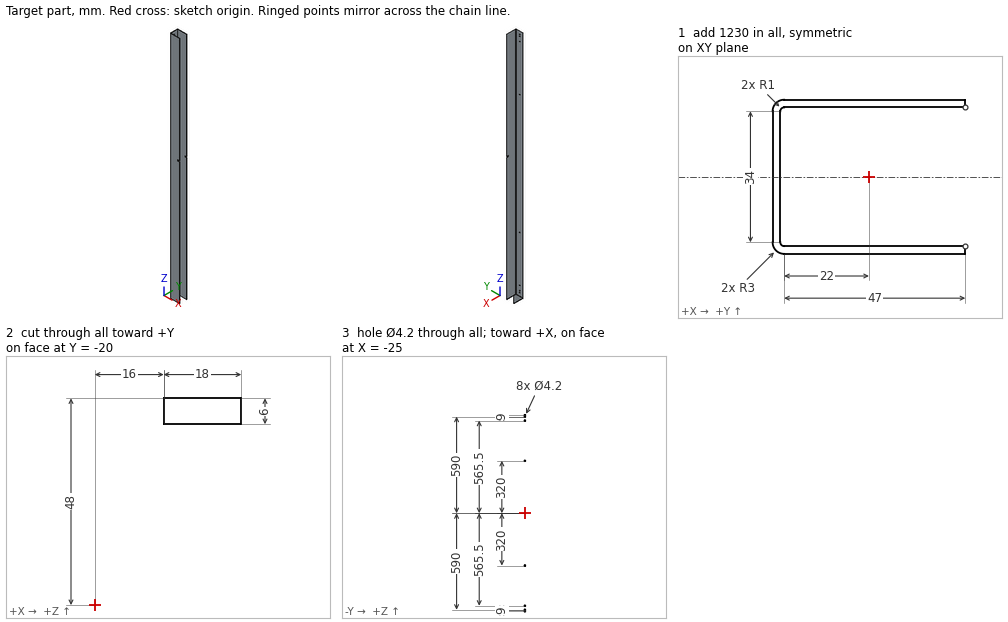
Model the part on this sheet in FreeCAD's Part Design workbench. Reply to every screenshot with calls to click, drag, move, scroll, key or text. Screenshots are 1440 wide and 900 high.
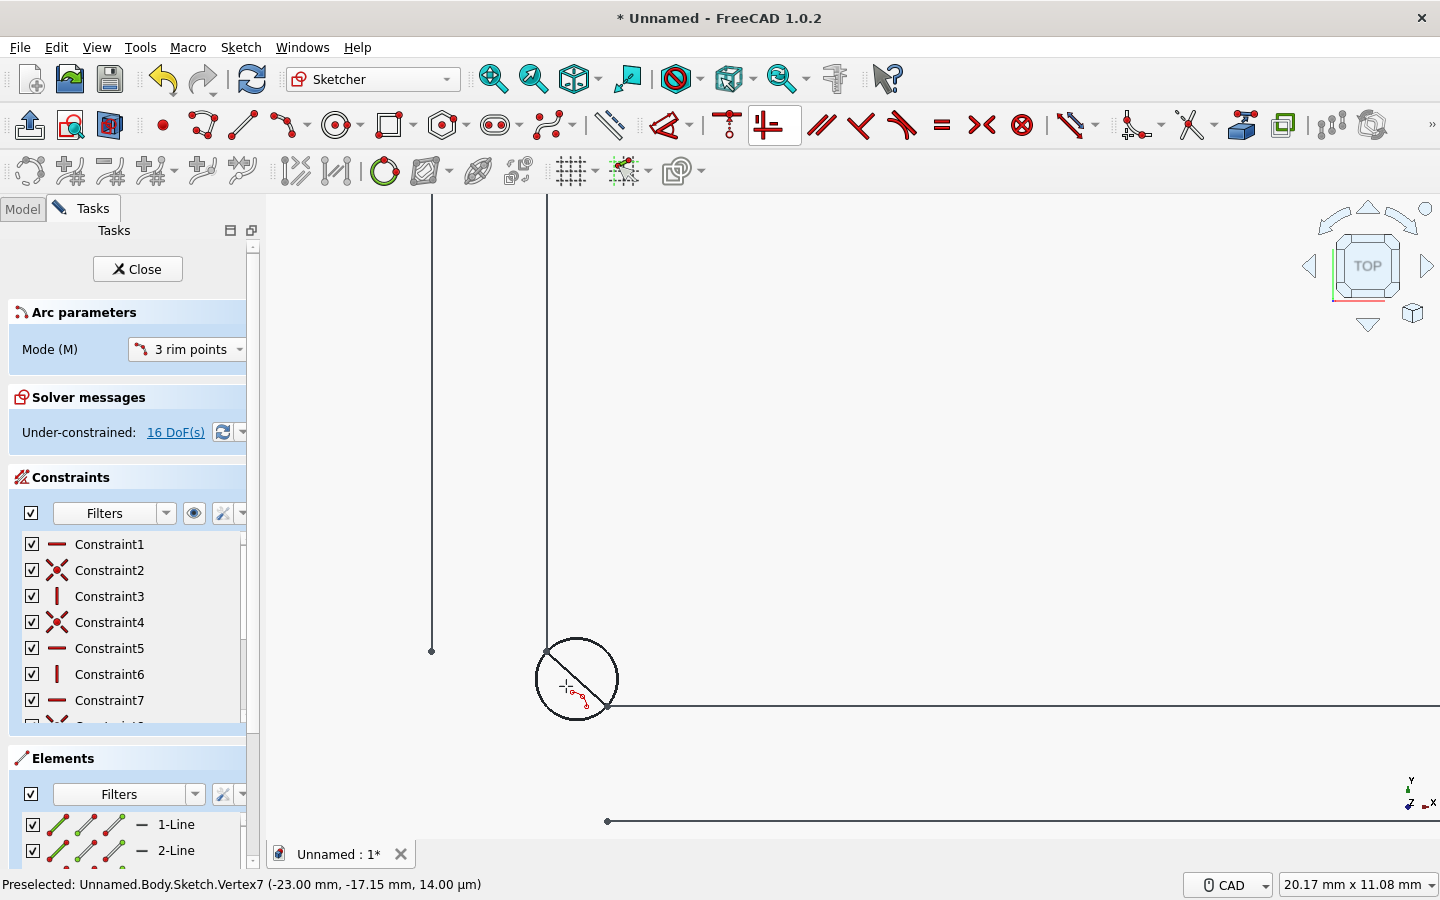
click(564, 685)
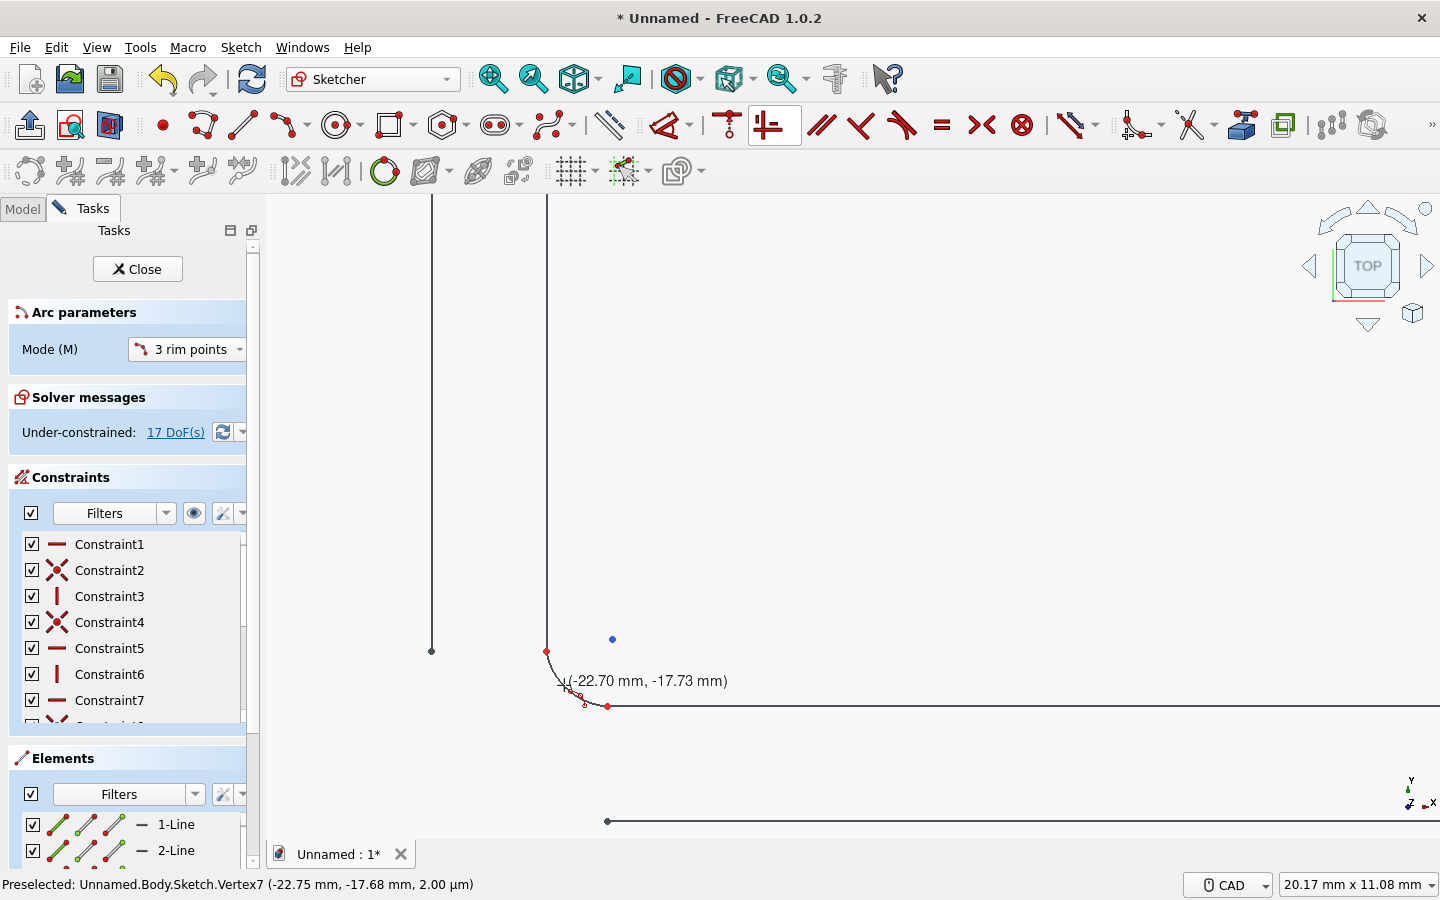
scroll(566, 687, down, 9)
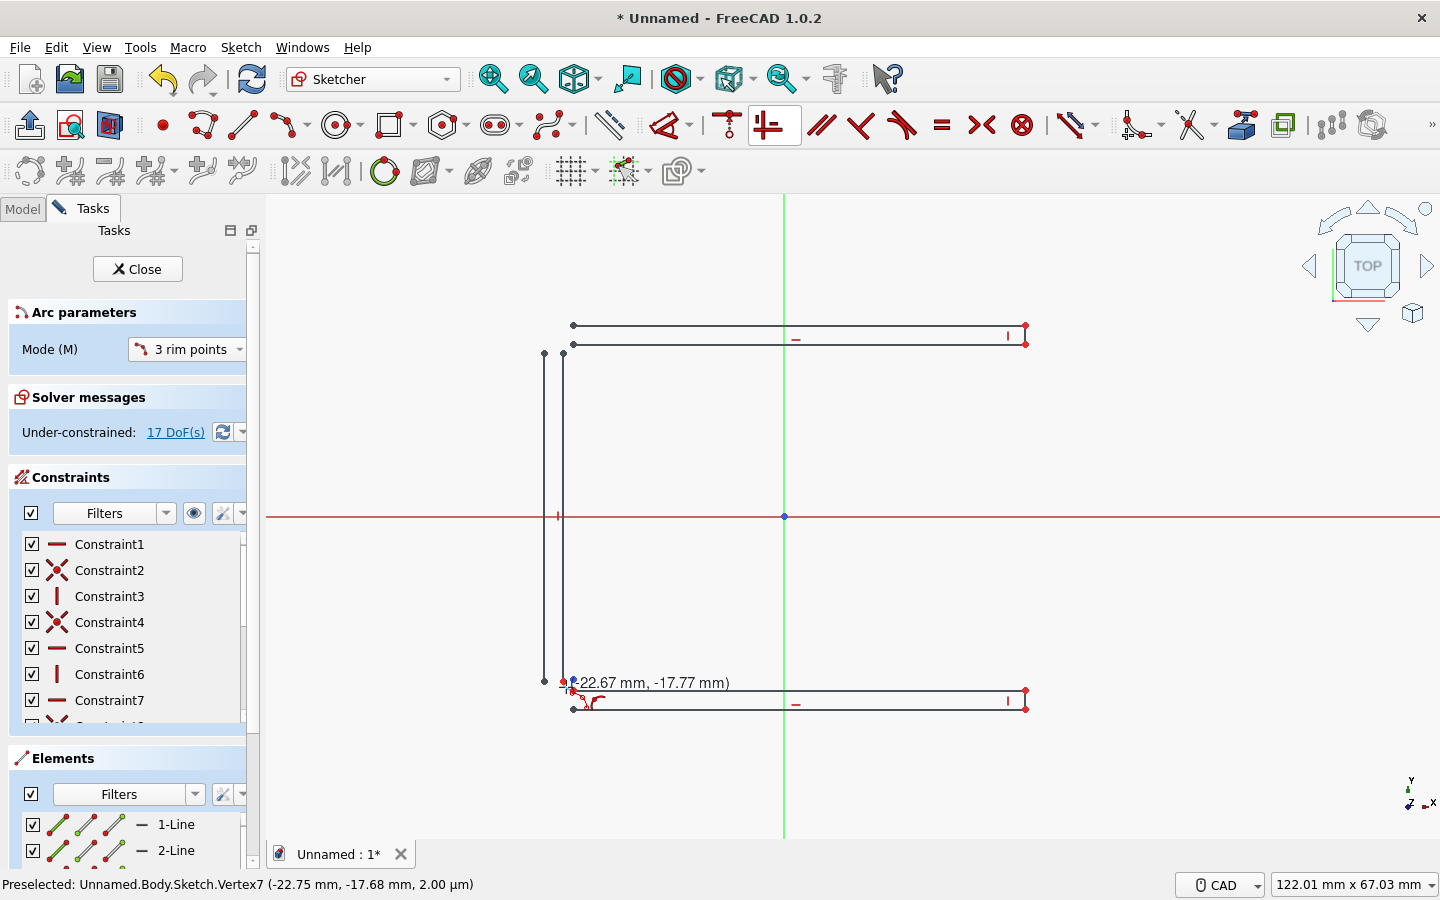
click(563, 354)
click(573, 345)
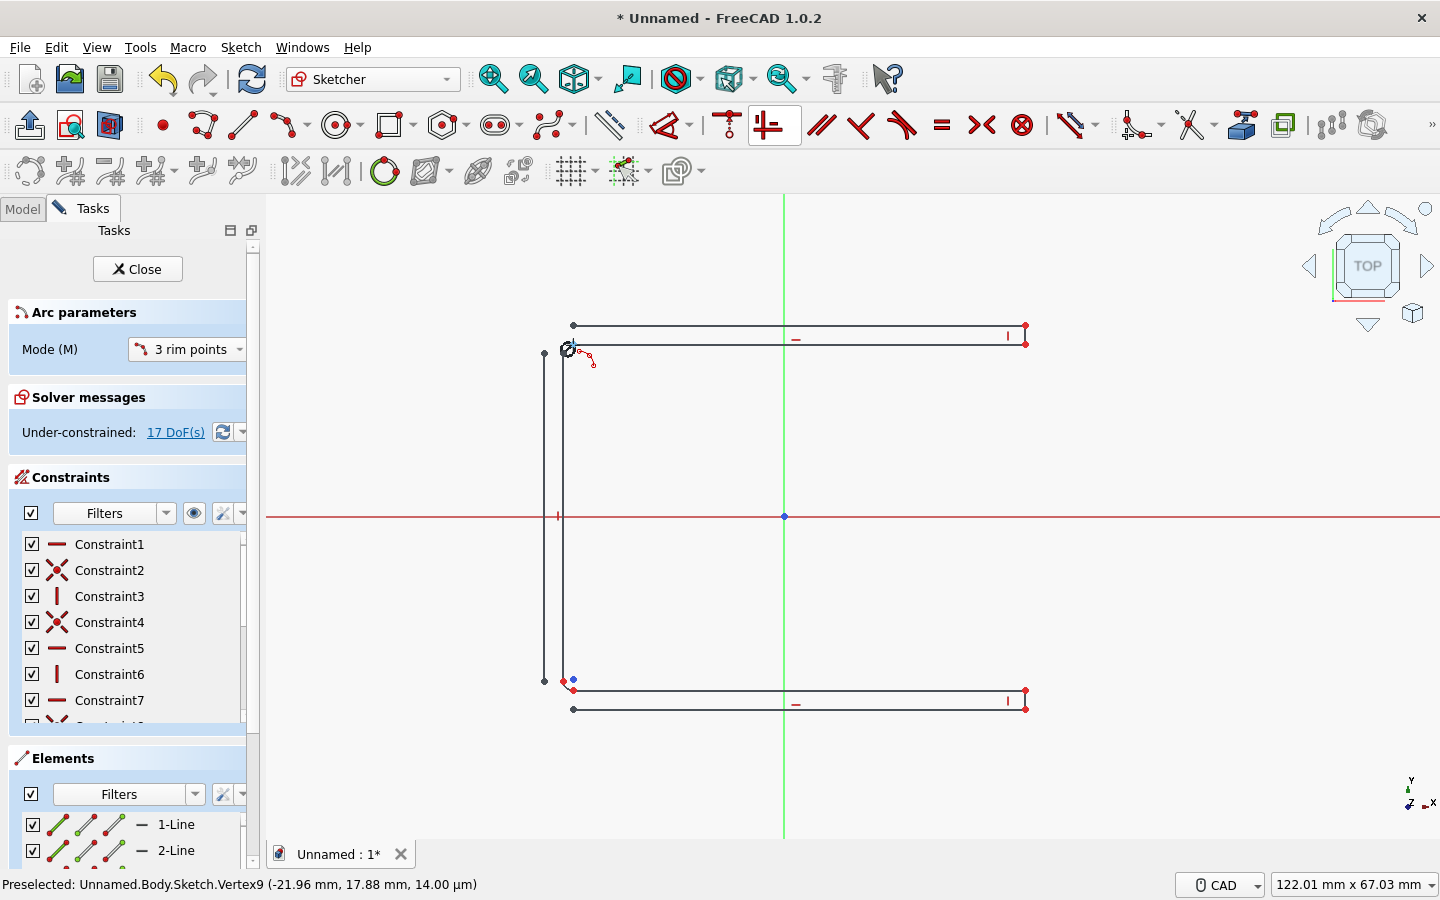
scroll(566, 346, up, 9)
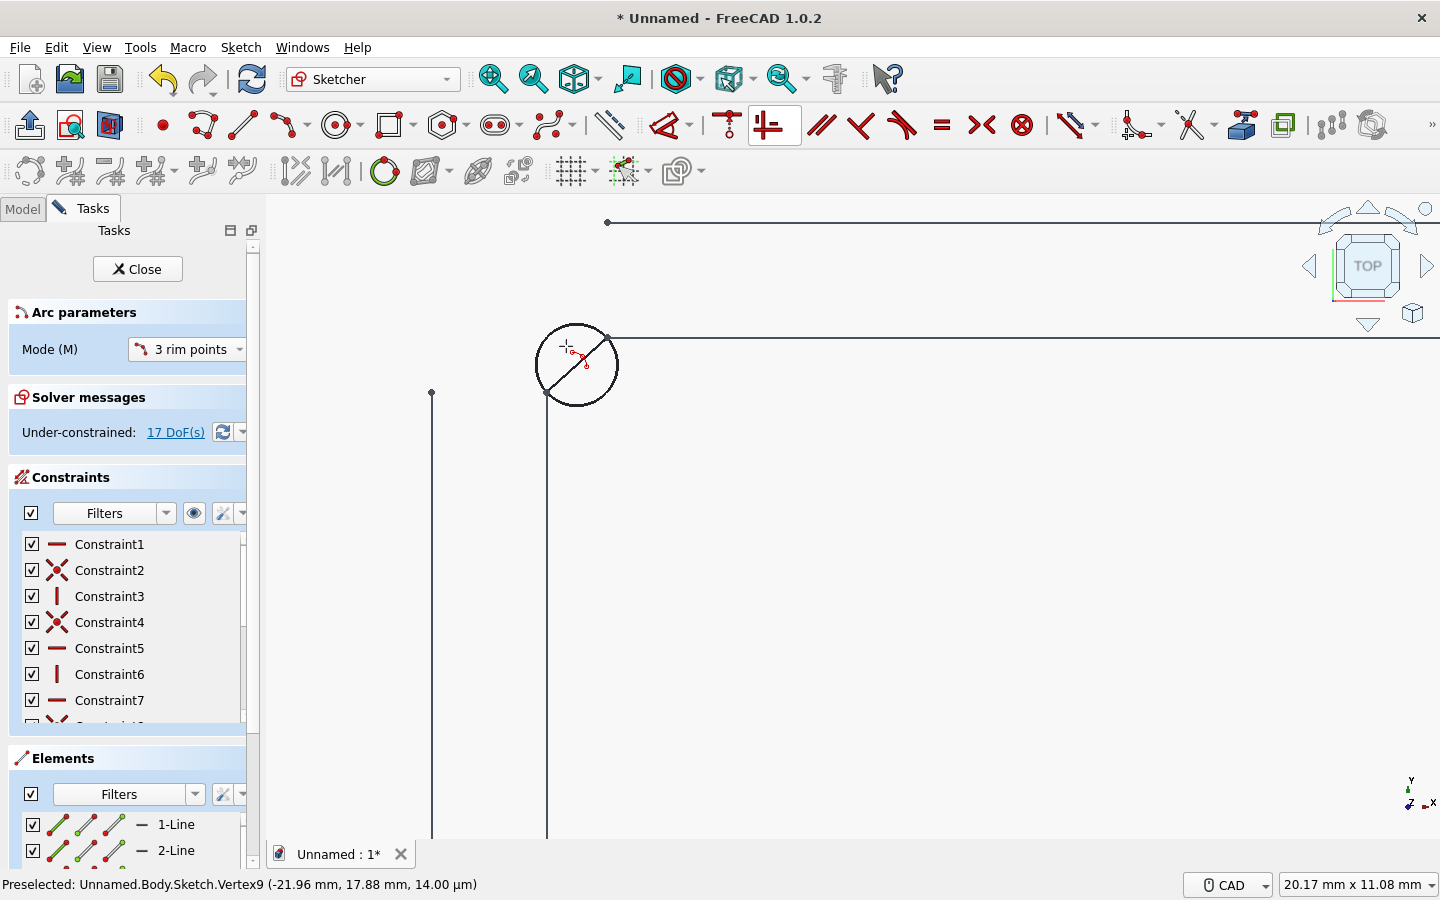
click(564, 348)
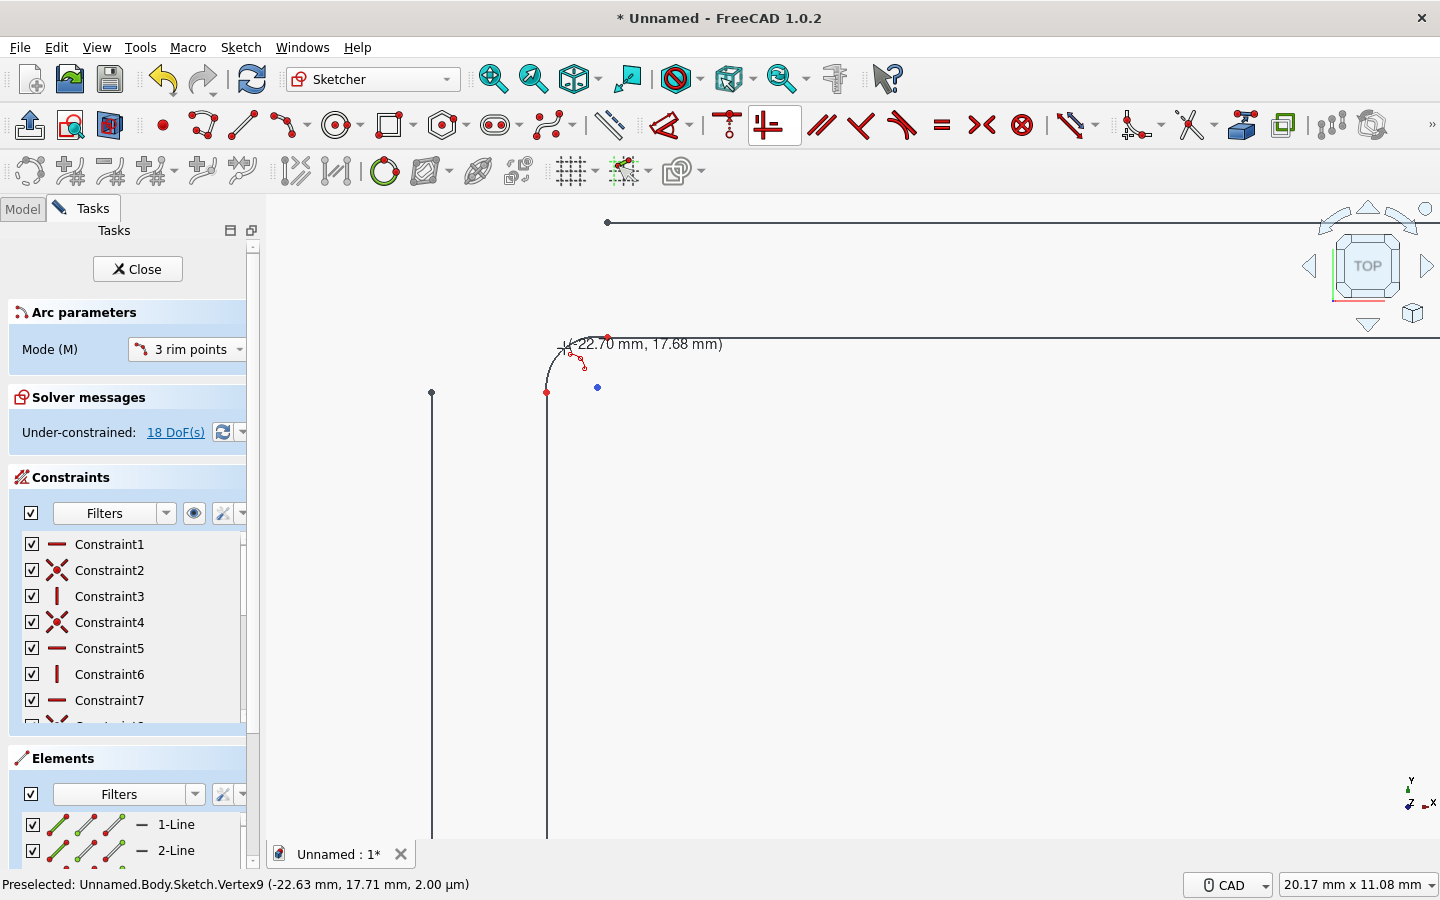
scroll(566, 346, down, 9)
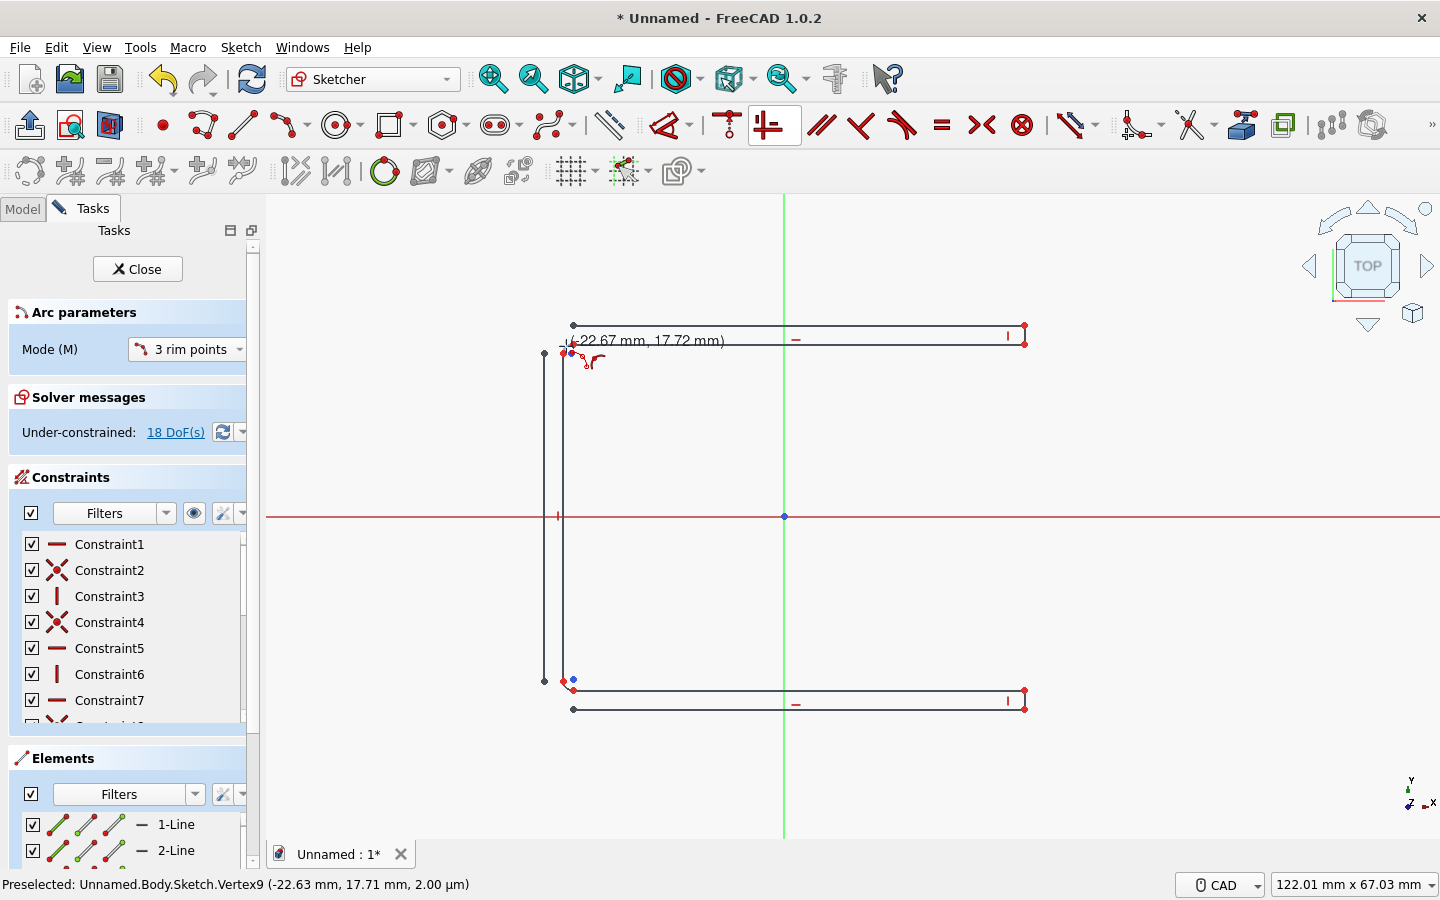
click(573, 326)
click(544, 354)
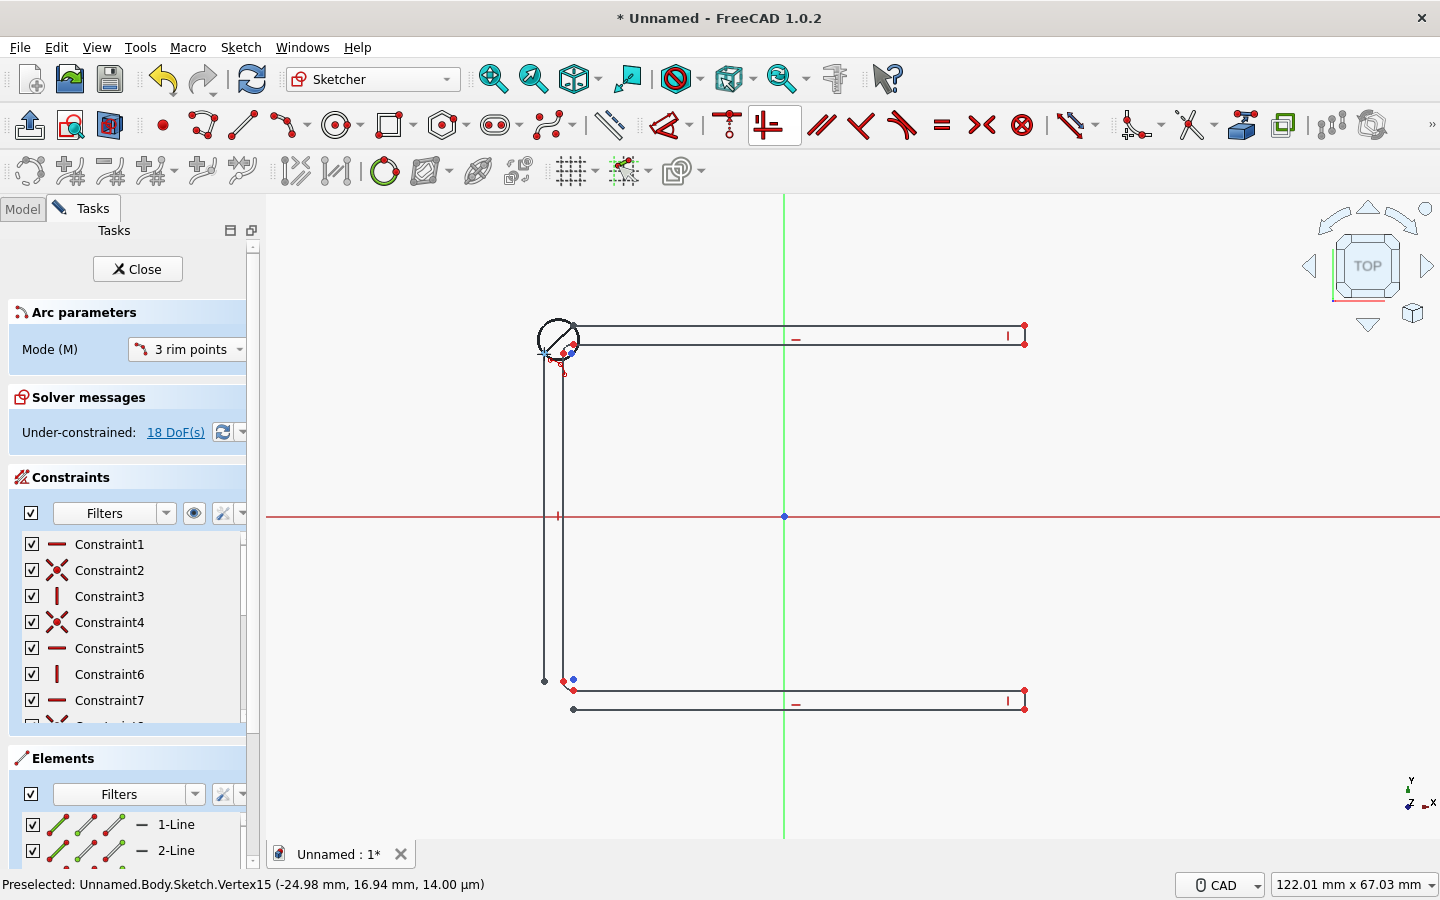
scroll(552, 333, up, 4)